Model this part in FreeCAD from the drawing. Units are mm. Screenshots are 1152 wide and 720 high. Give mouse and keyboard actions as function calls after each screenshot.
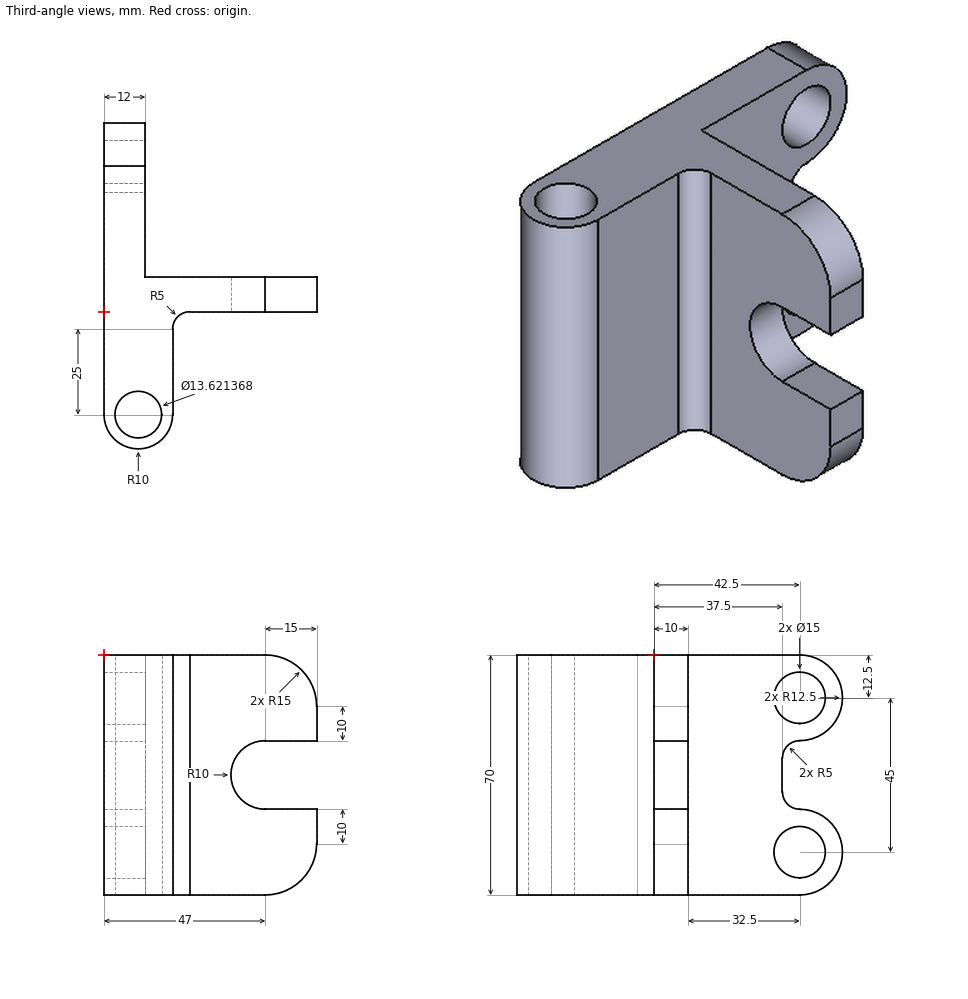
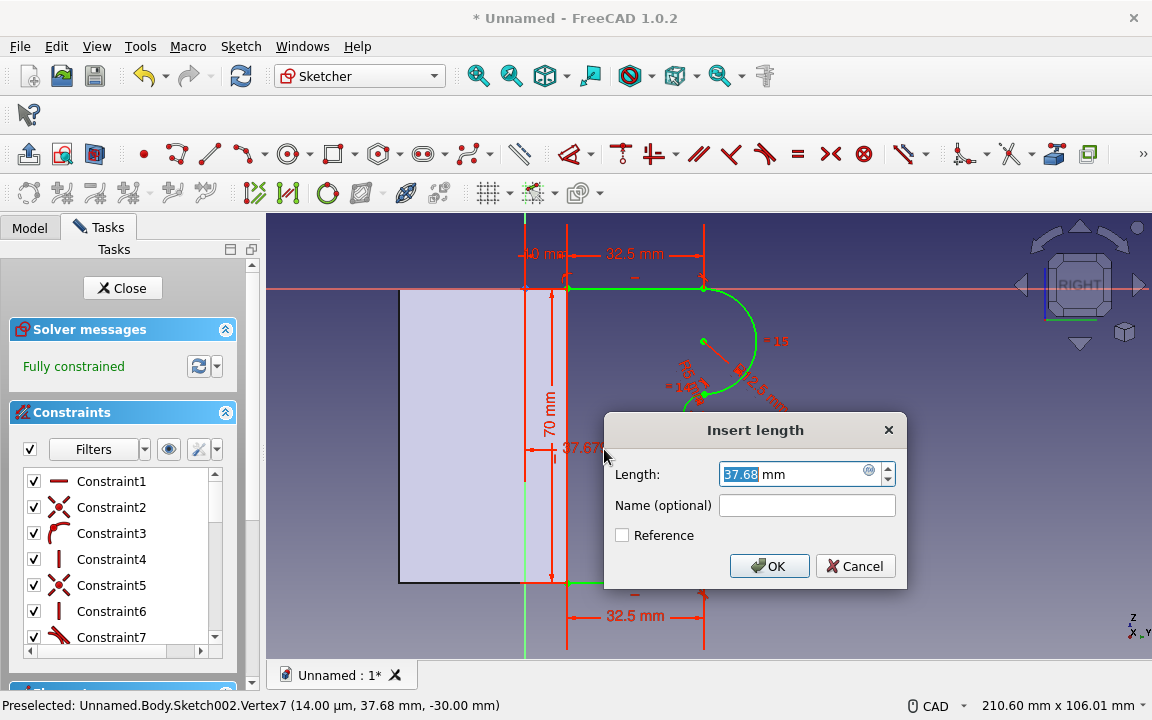
text(37.5)
key(Return)
key(Escape)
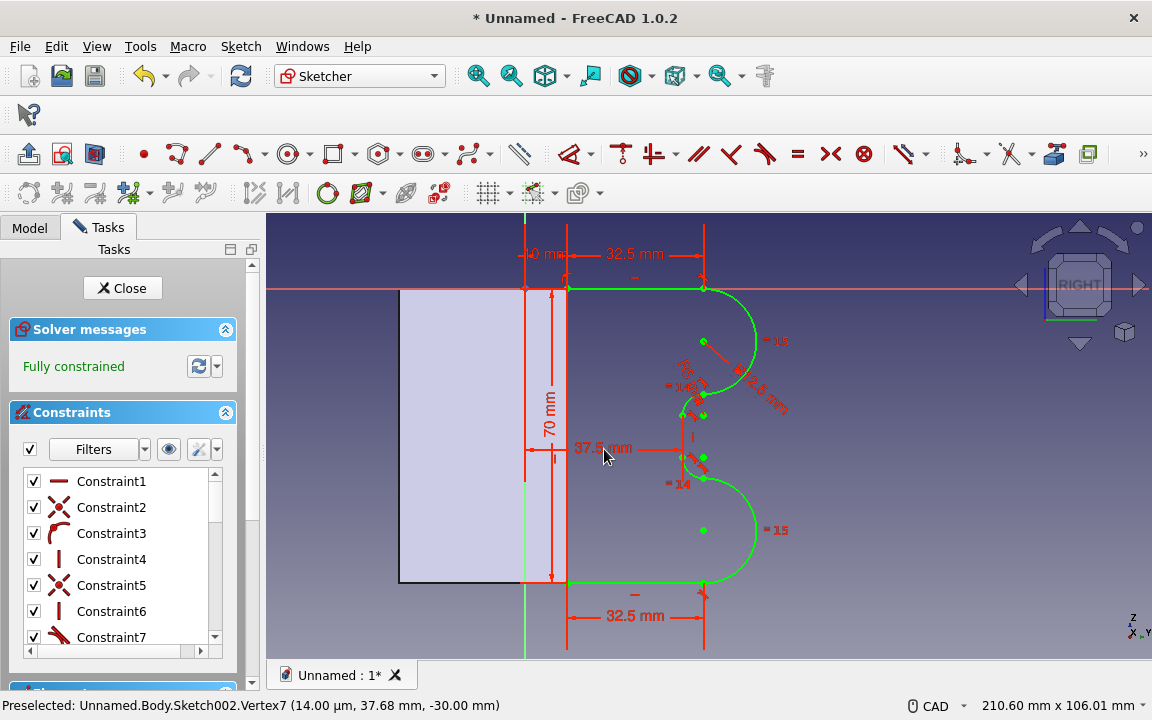
click(123, 288)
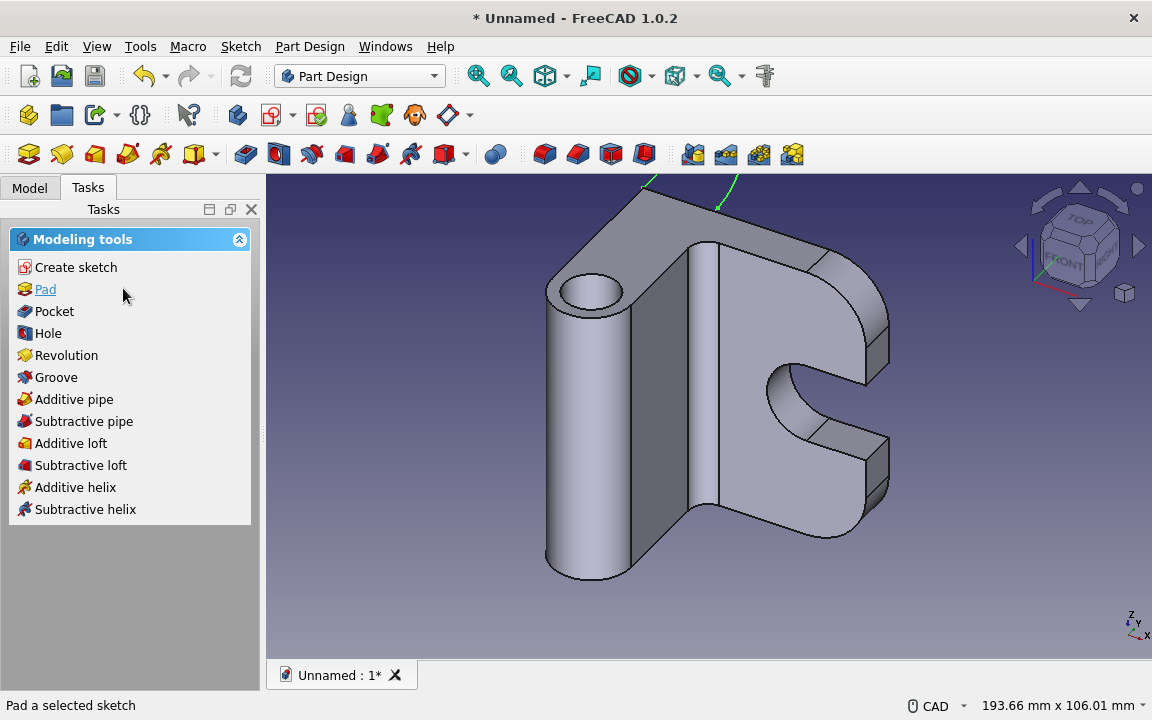
click(29, 154)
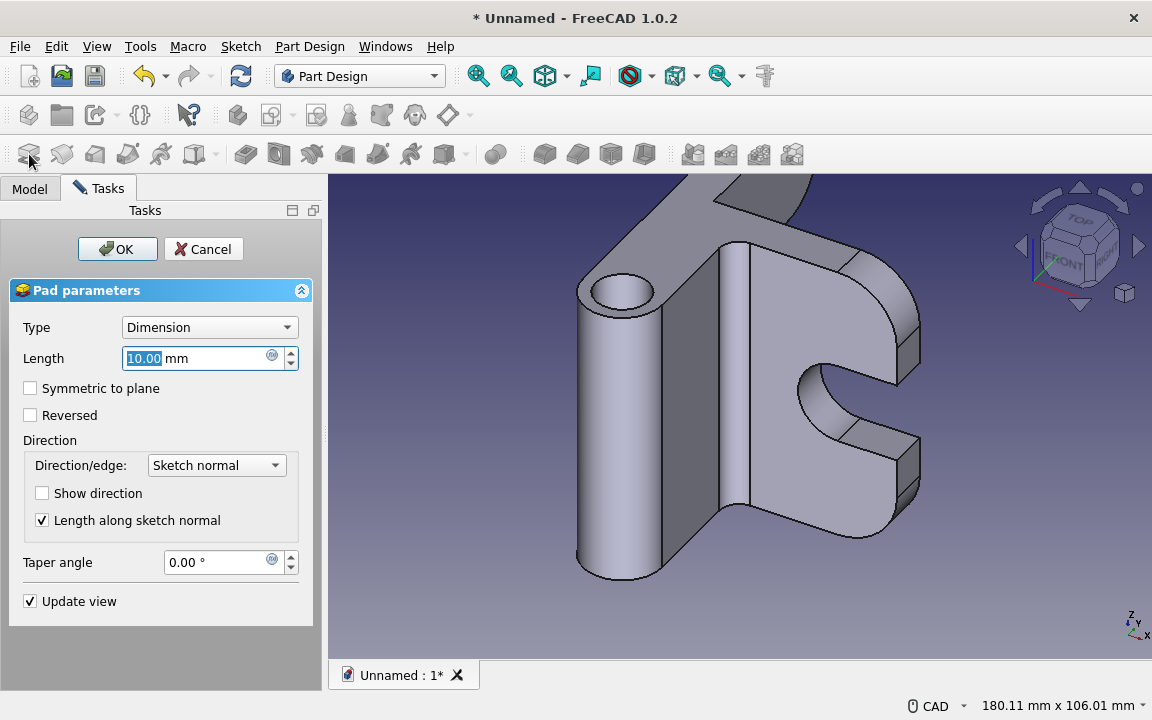
text(12)
key(Tab)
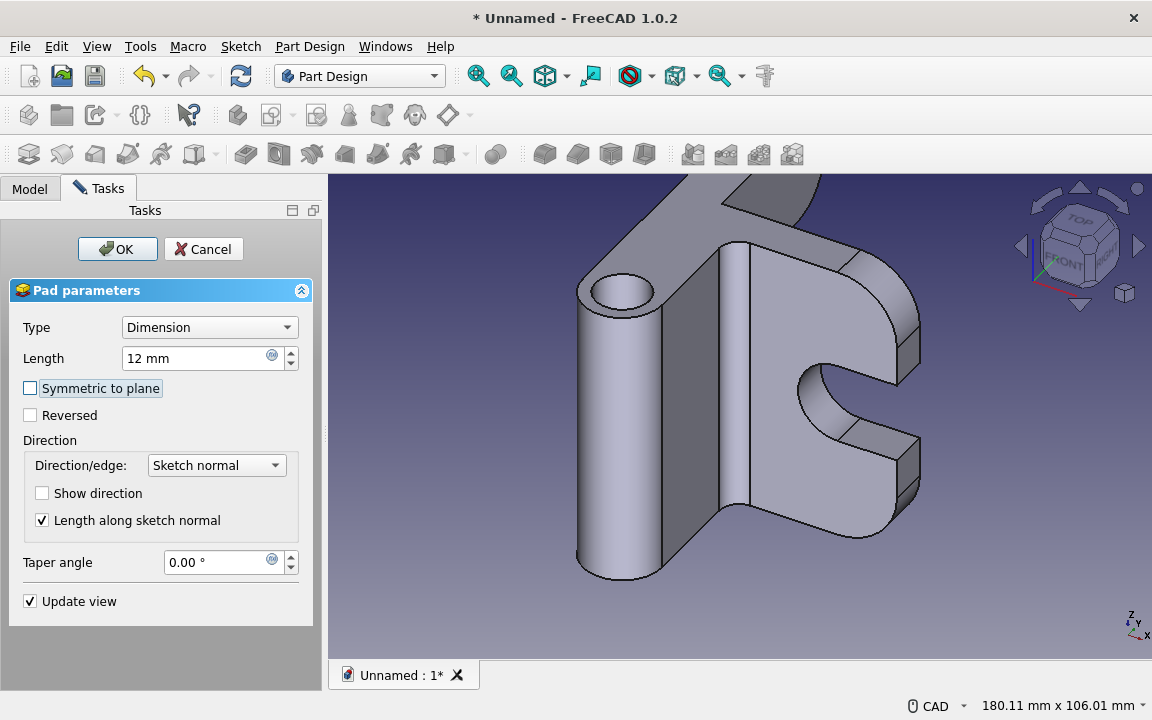
click(118, 249)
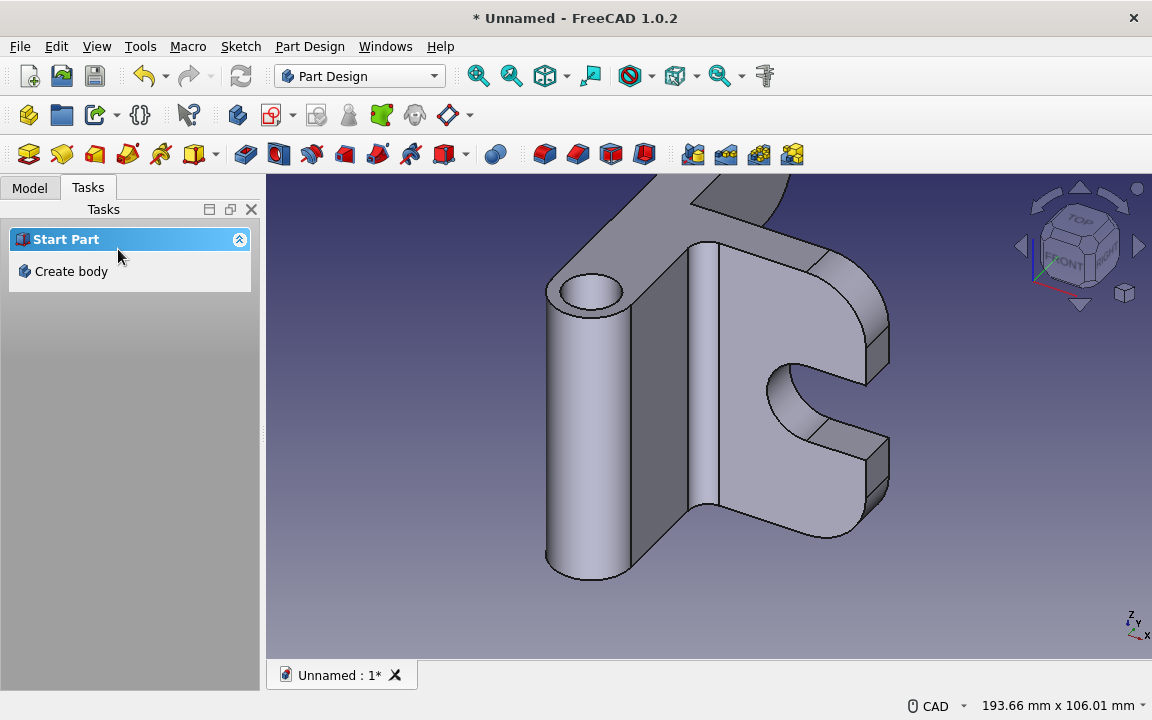
key(v)
key(f)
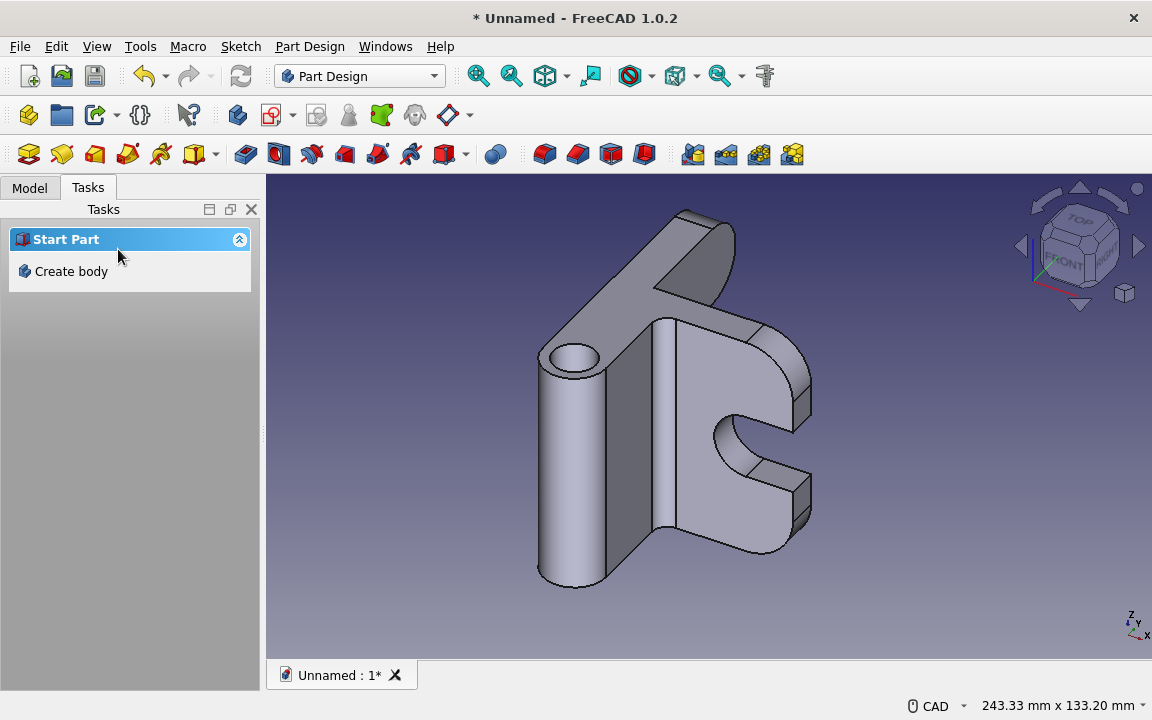
click(695, 291)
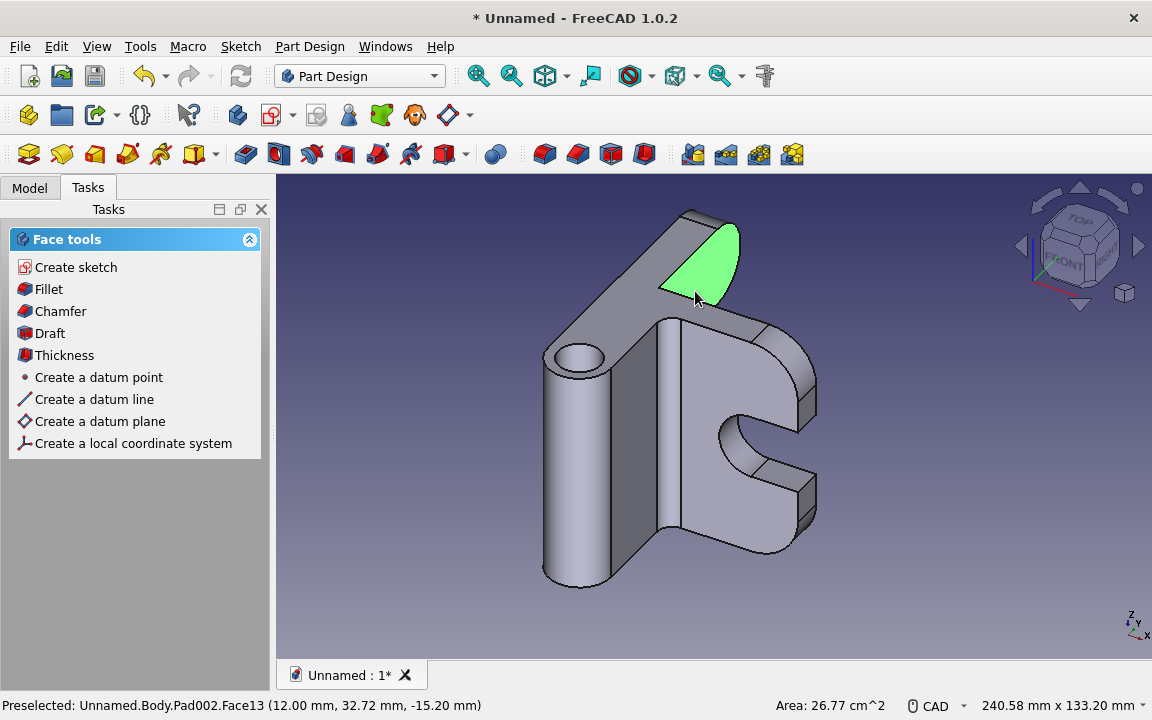
click(270, 116)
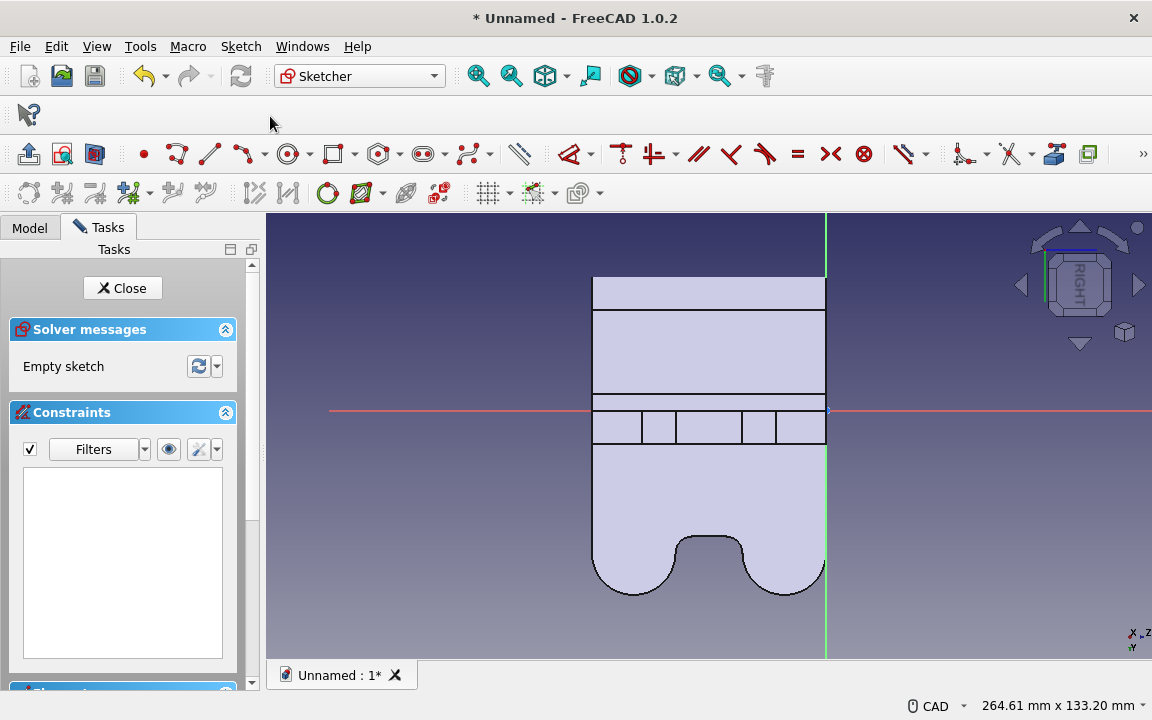
scroll(874, 614, up, 2)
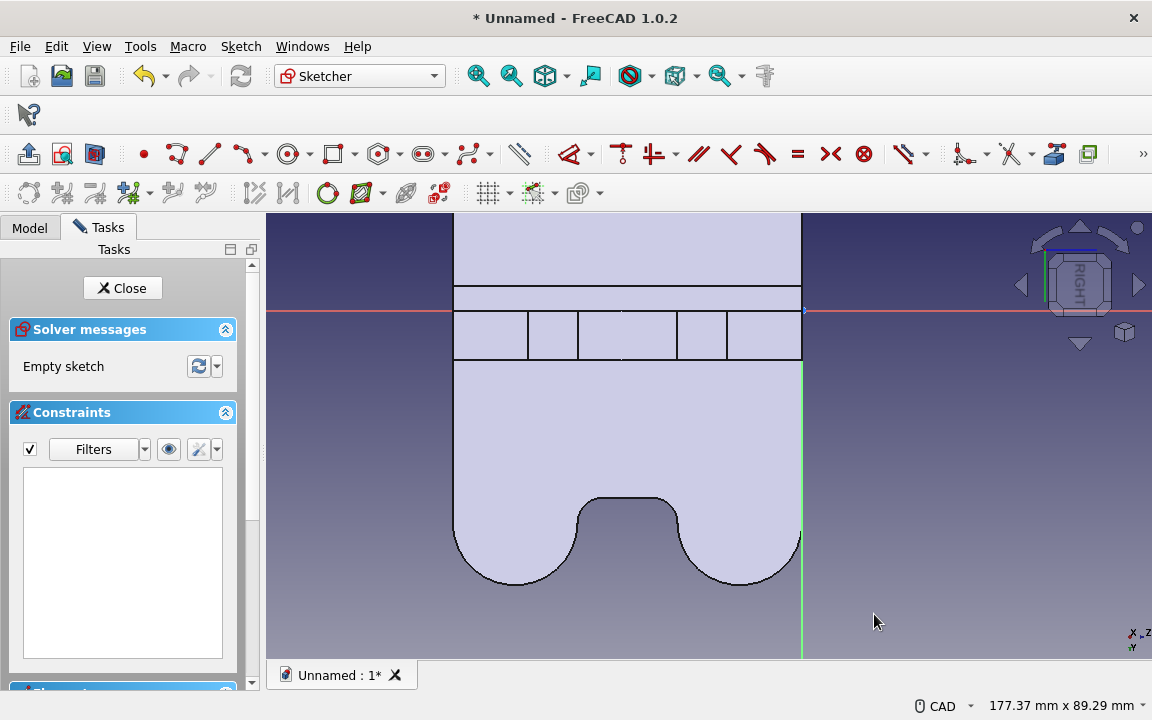
key(g)
key(c)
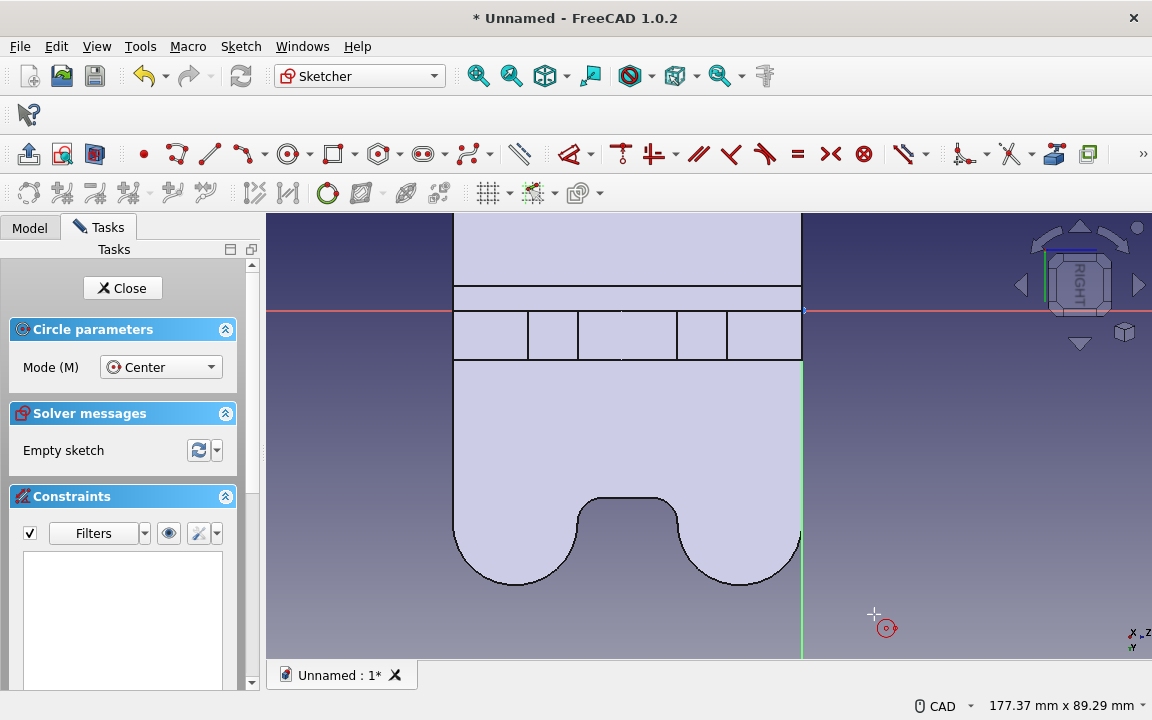
click(740, 523)
move(766, 496)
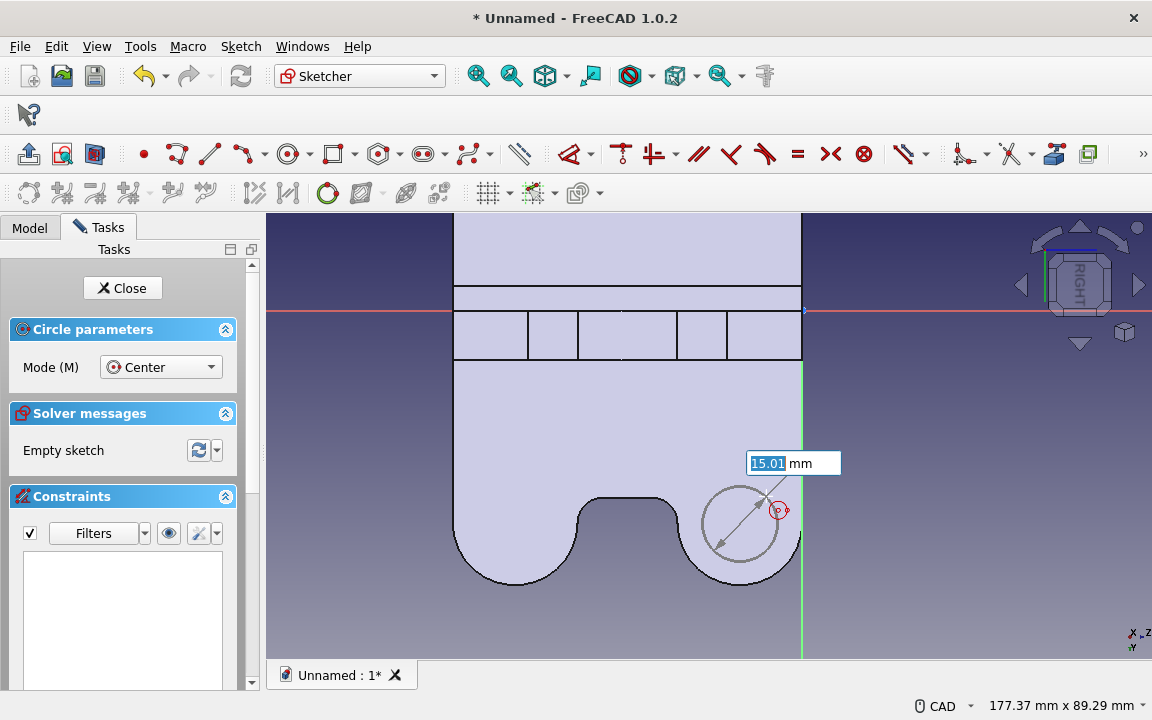
text(15)
key(Return)